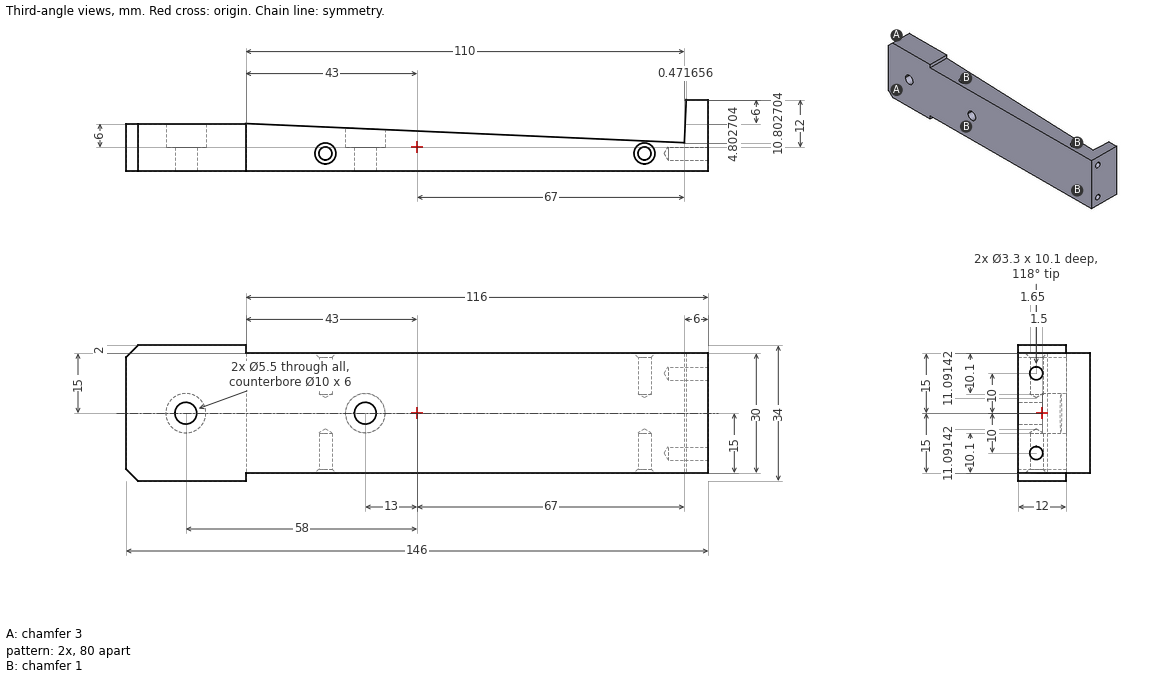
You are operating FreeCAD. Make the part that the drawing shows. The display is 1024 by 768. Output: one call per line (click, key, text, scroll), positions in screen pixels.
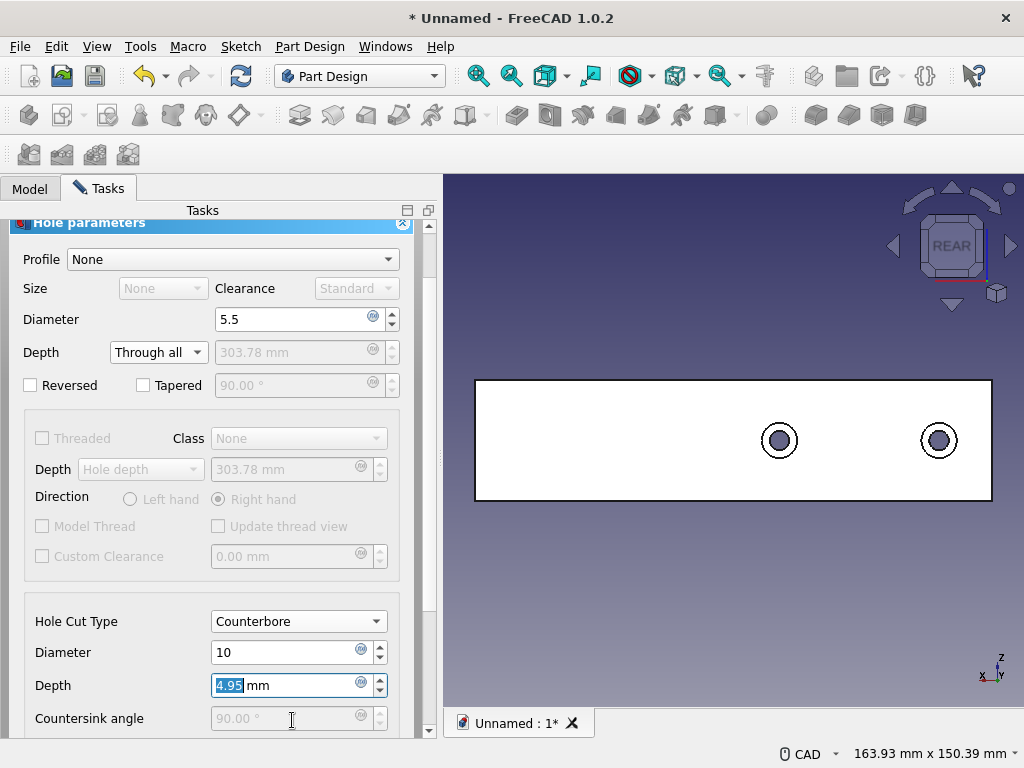
text(6)
key(Tab)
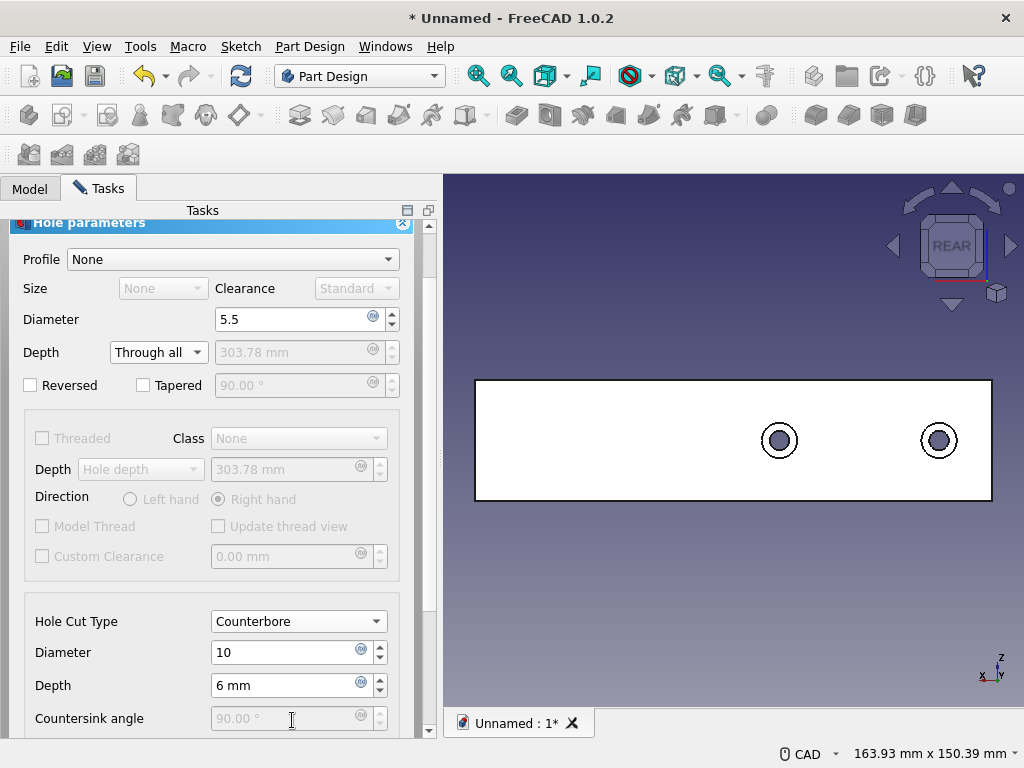
scroll(429, 479, up, 2)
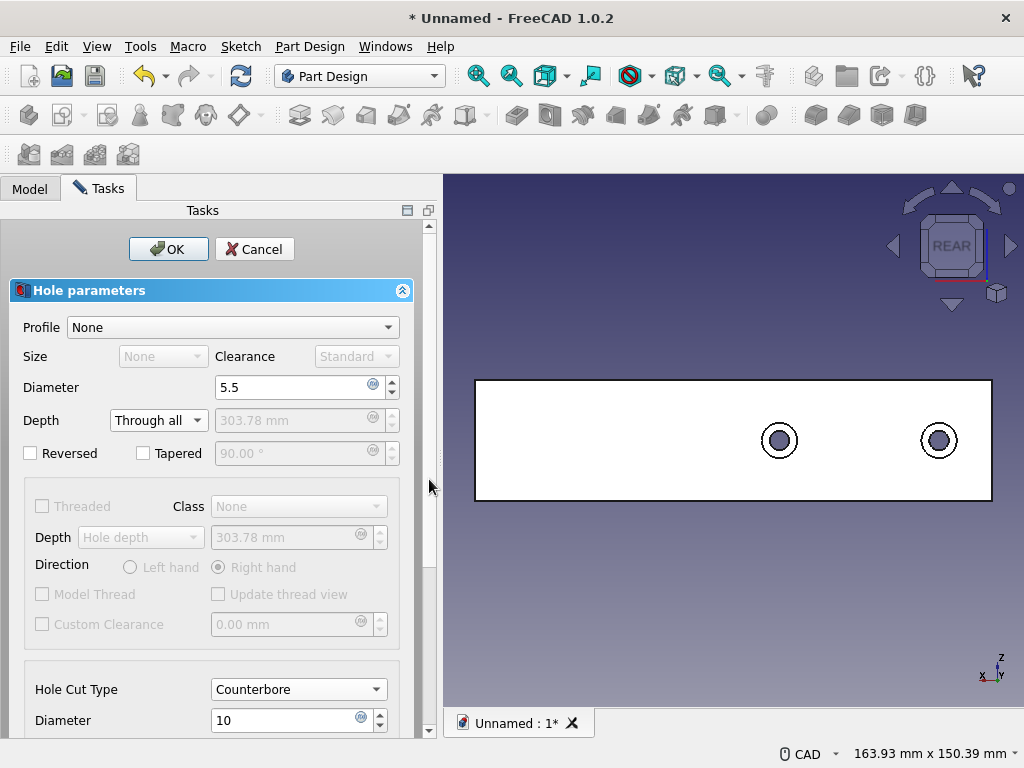
click(169, 249)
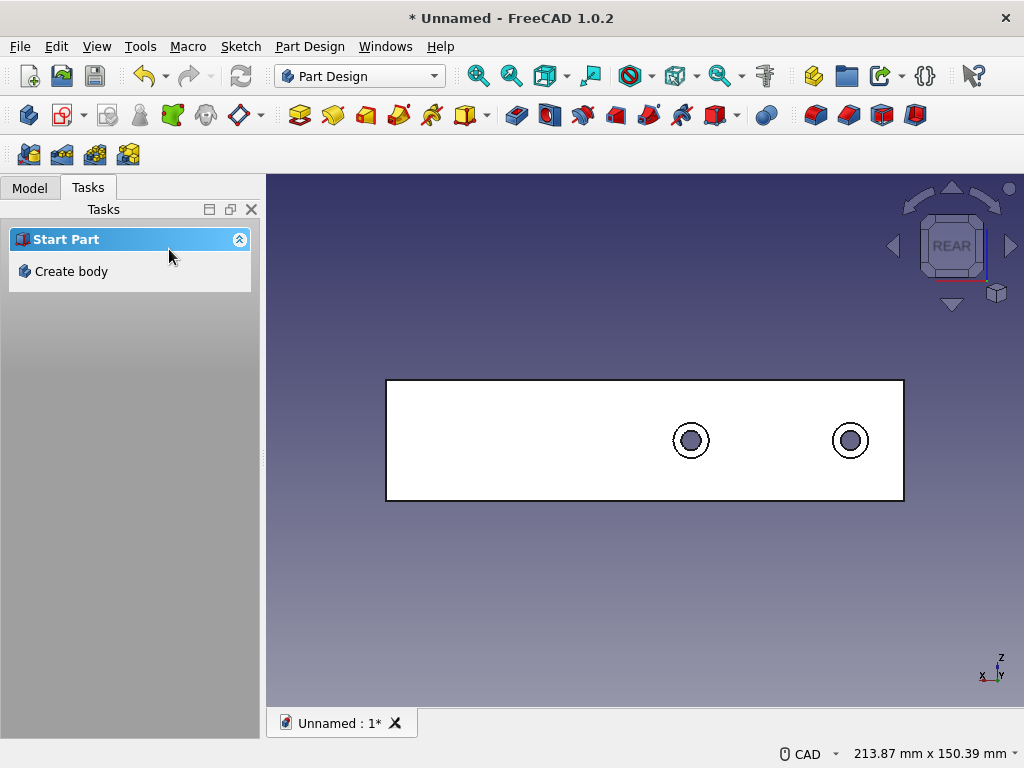
key(0)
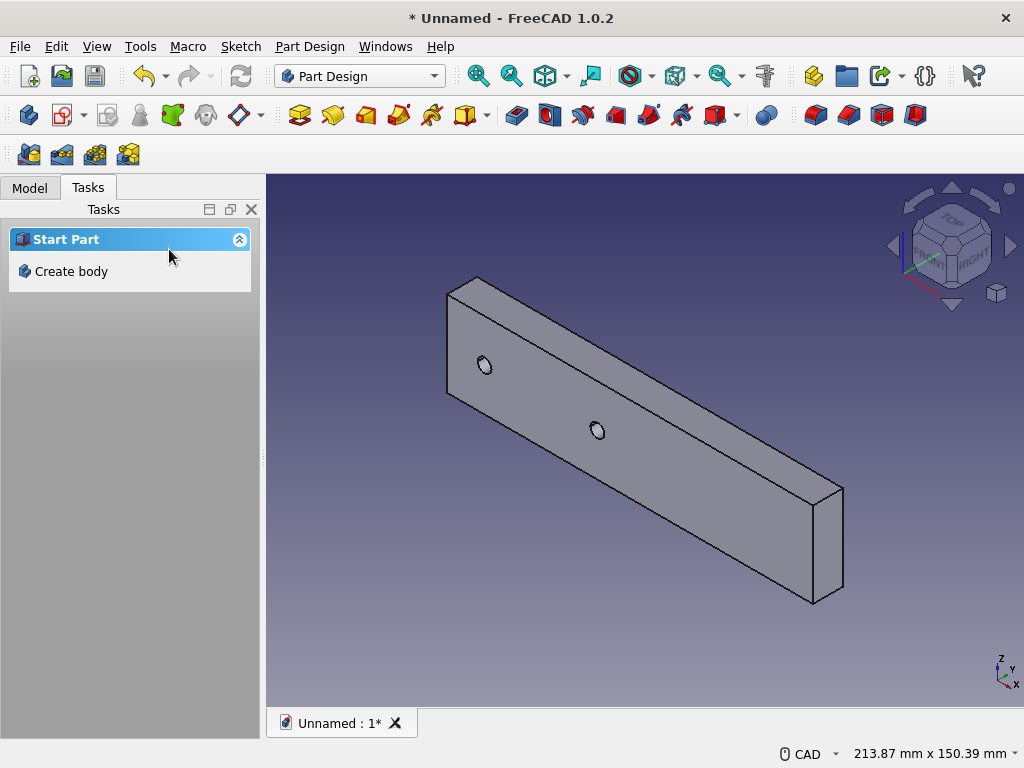
click(828, 517)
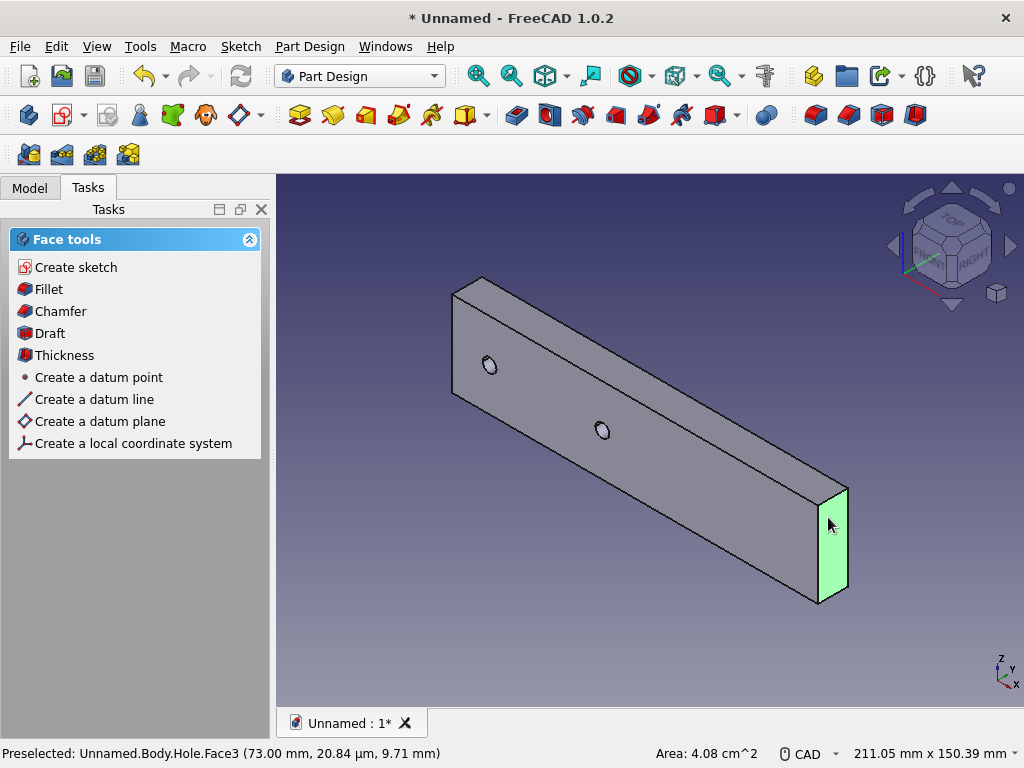
click(62, 116)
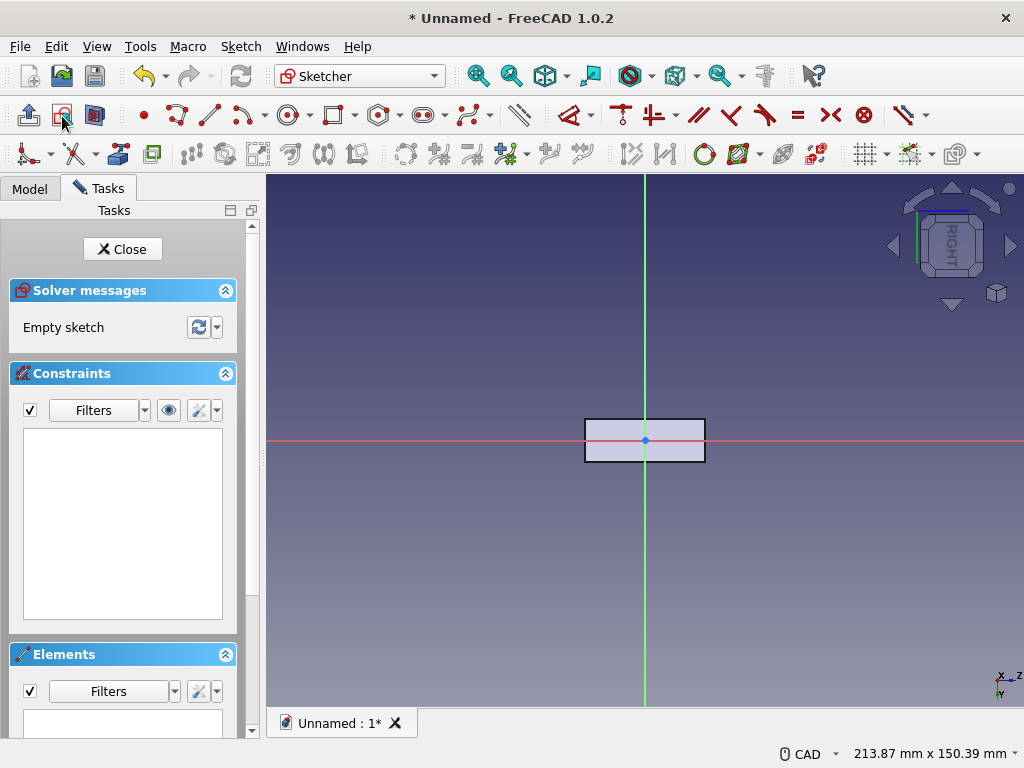
scroll(662, 434, up, 8)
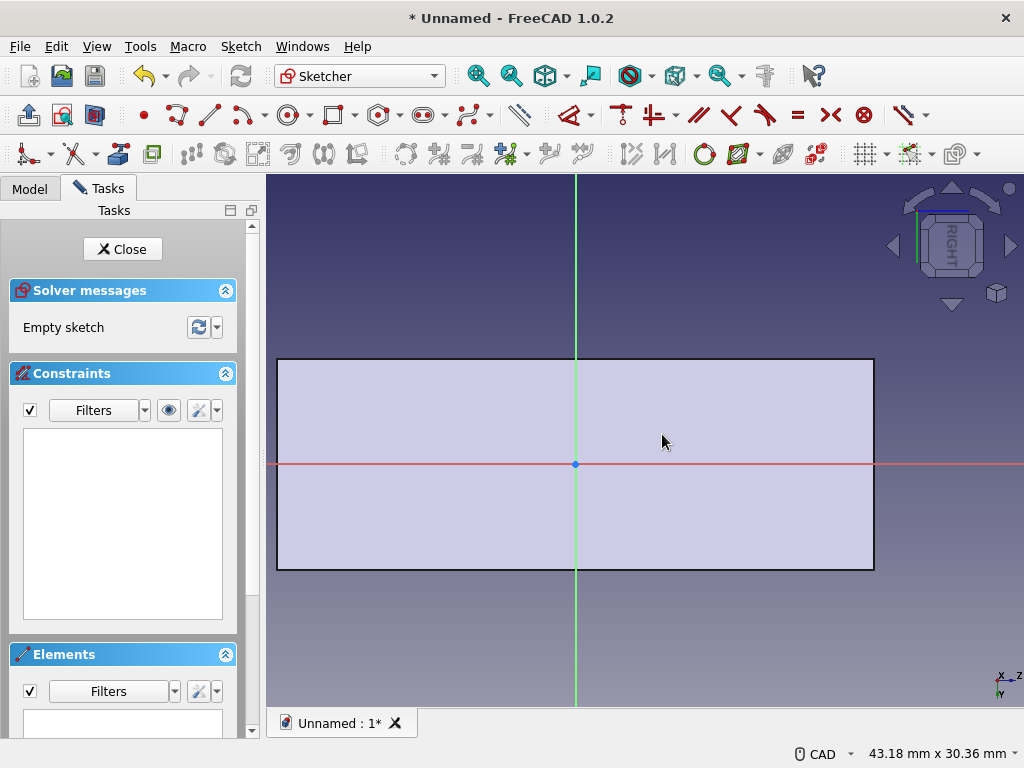
click(288, 116)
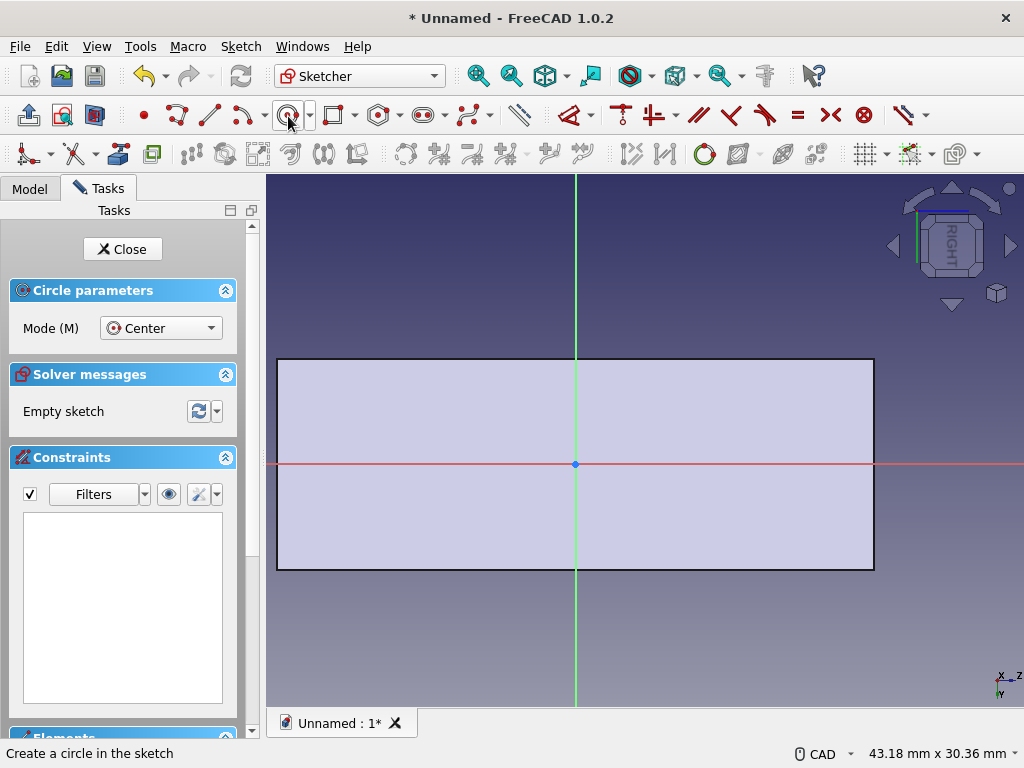
click(751, 438)
move(772, 417)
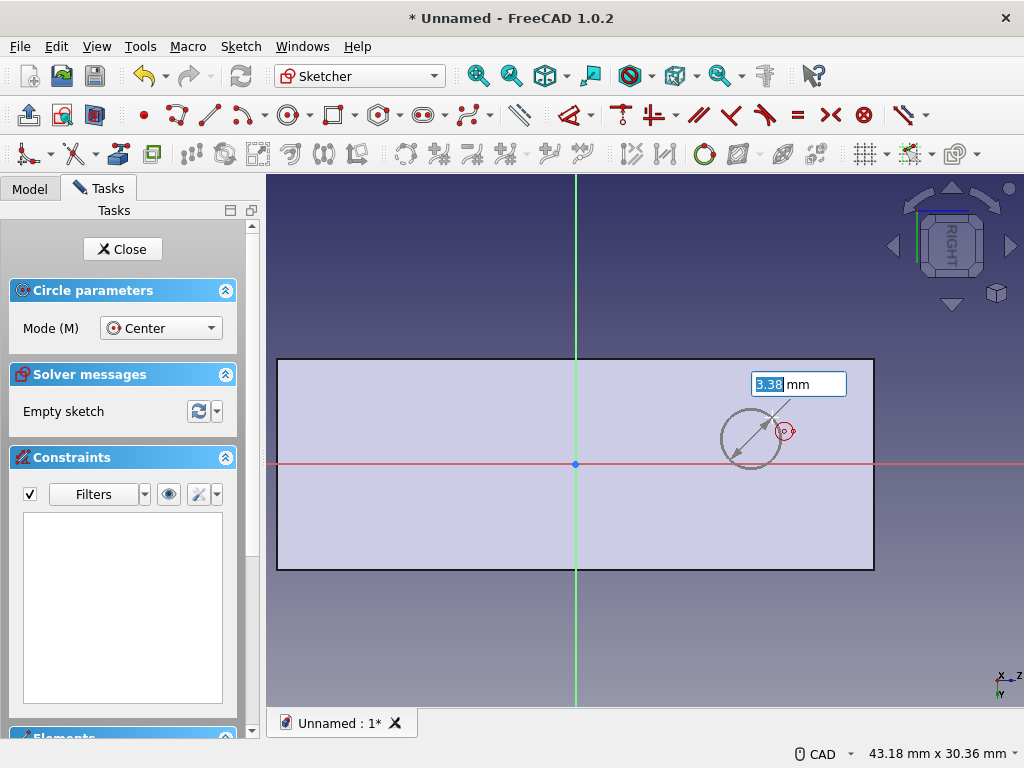
text(3.3)
key(Return)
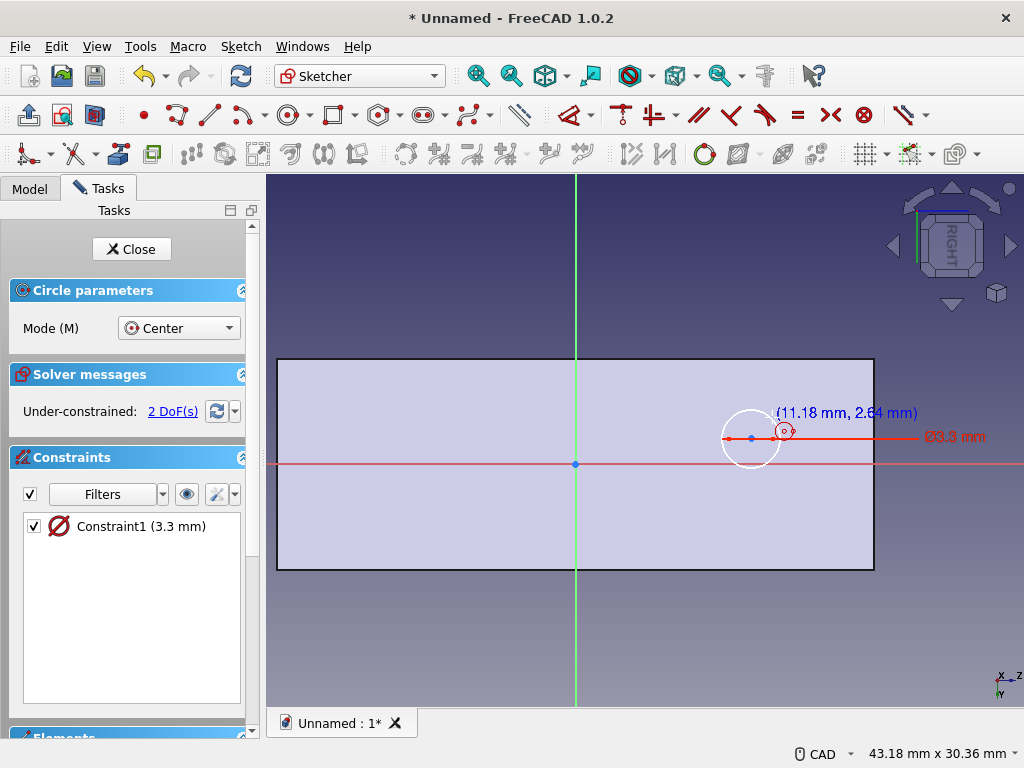
click(400, 438)
move(421, 417)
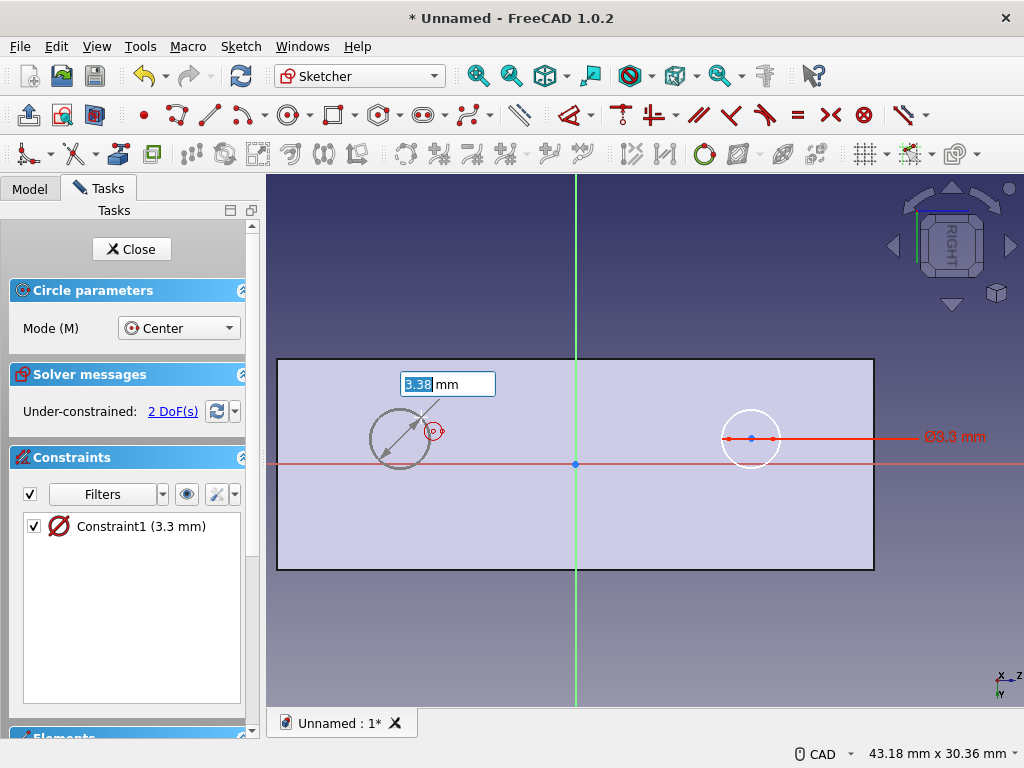
text(3.3)
key(Return)
key(Escape)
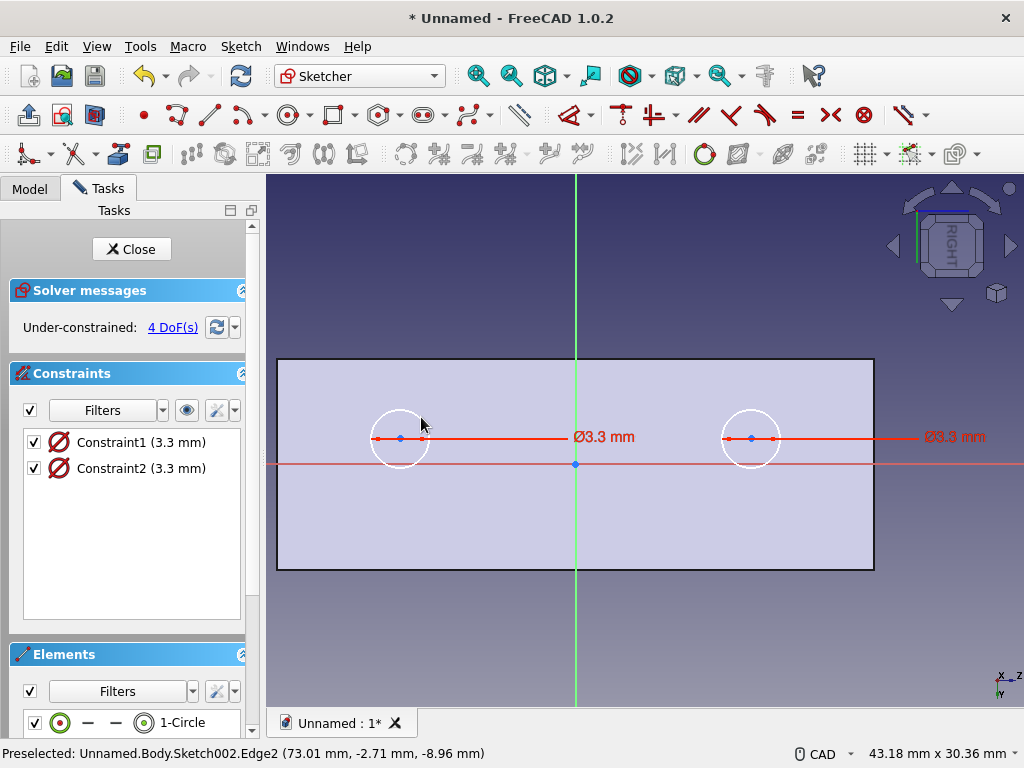
click(751, 439)